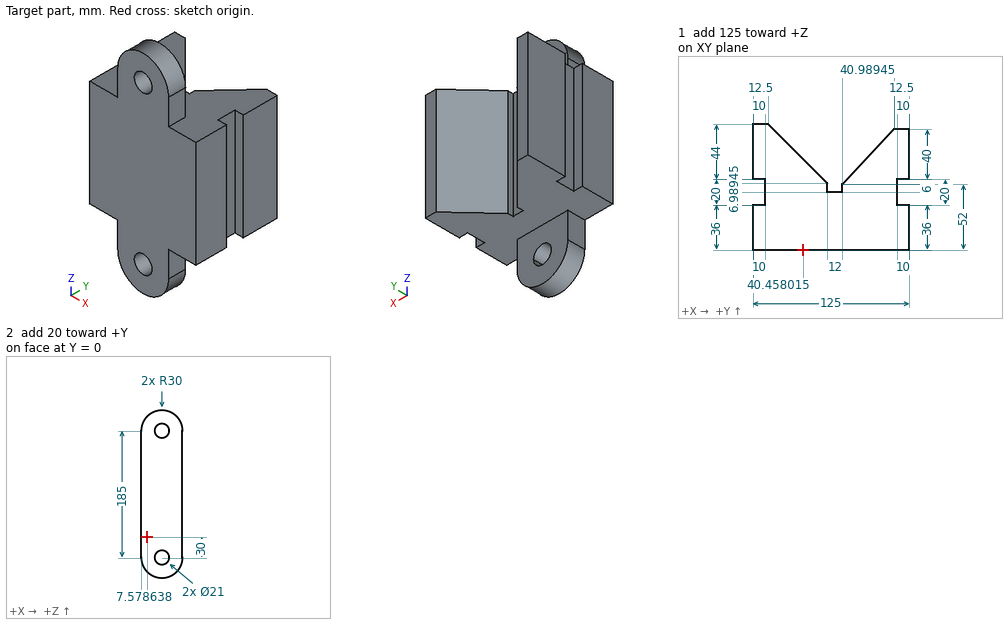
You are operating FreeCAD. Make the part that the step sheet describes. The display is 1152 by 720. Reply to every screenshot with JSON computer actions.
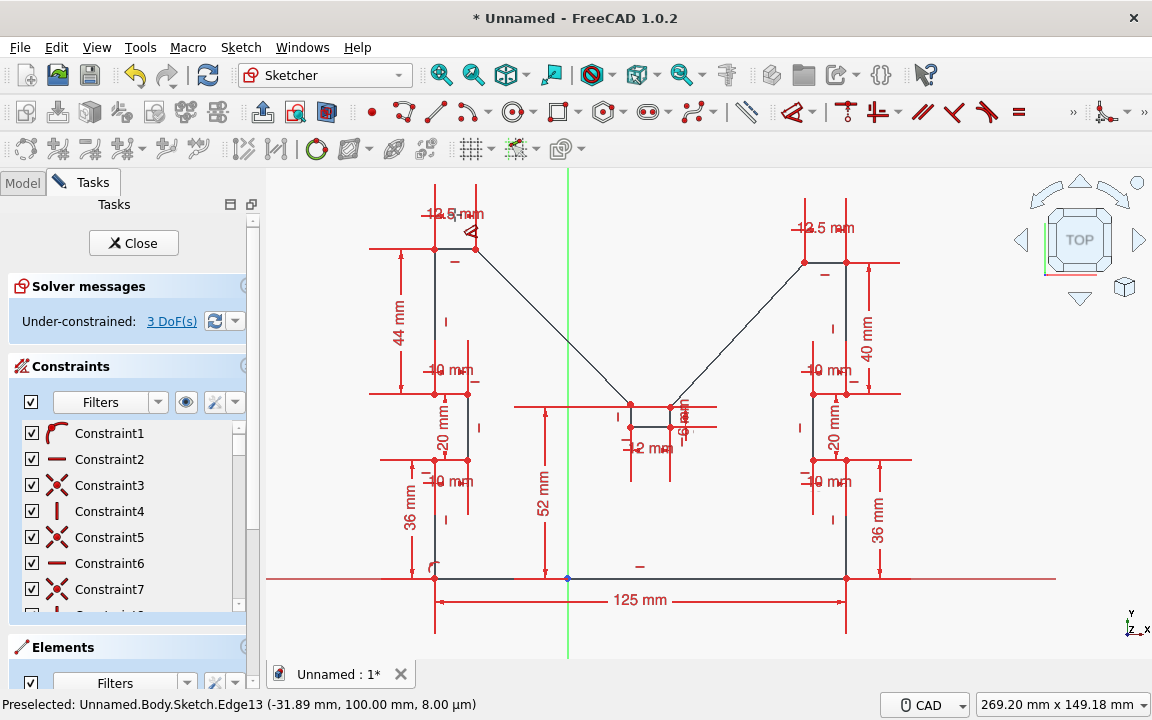
{"action": "scroll", "coordinate": [631, 416], "scroll_direction": "up", "scroll_amount": 3}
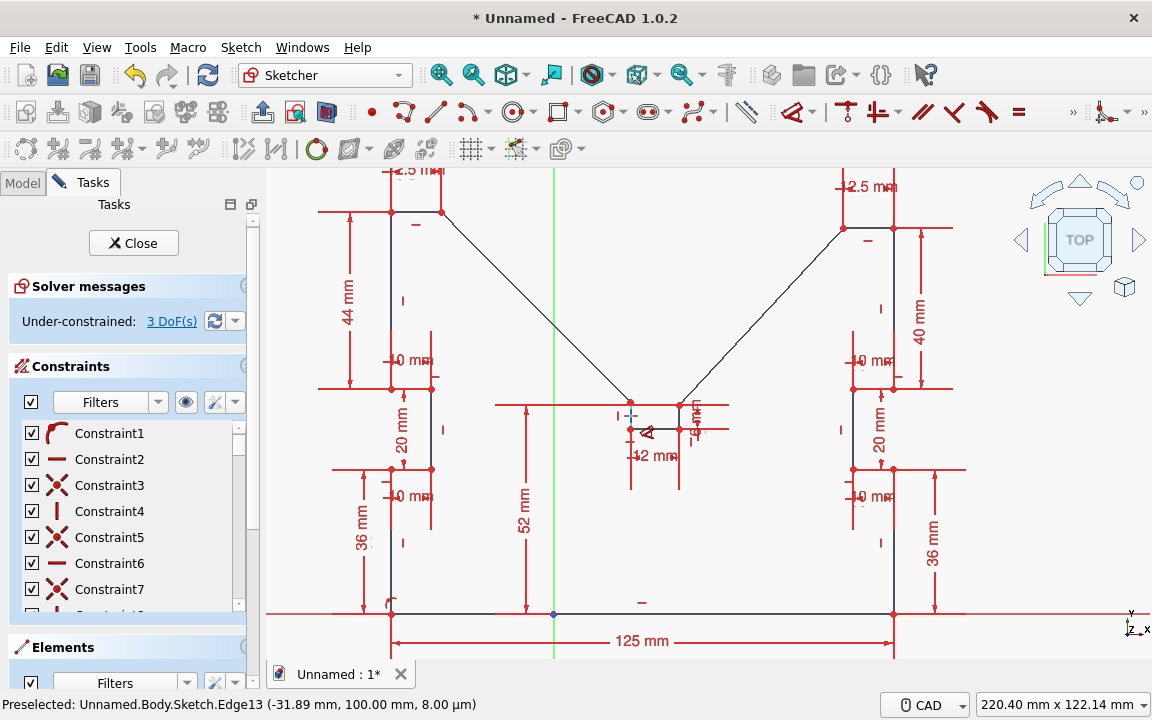
{"action": "left_click", "coordinate": [630, 416]}
{"action": "left_click", "coordinate": [596, 416]}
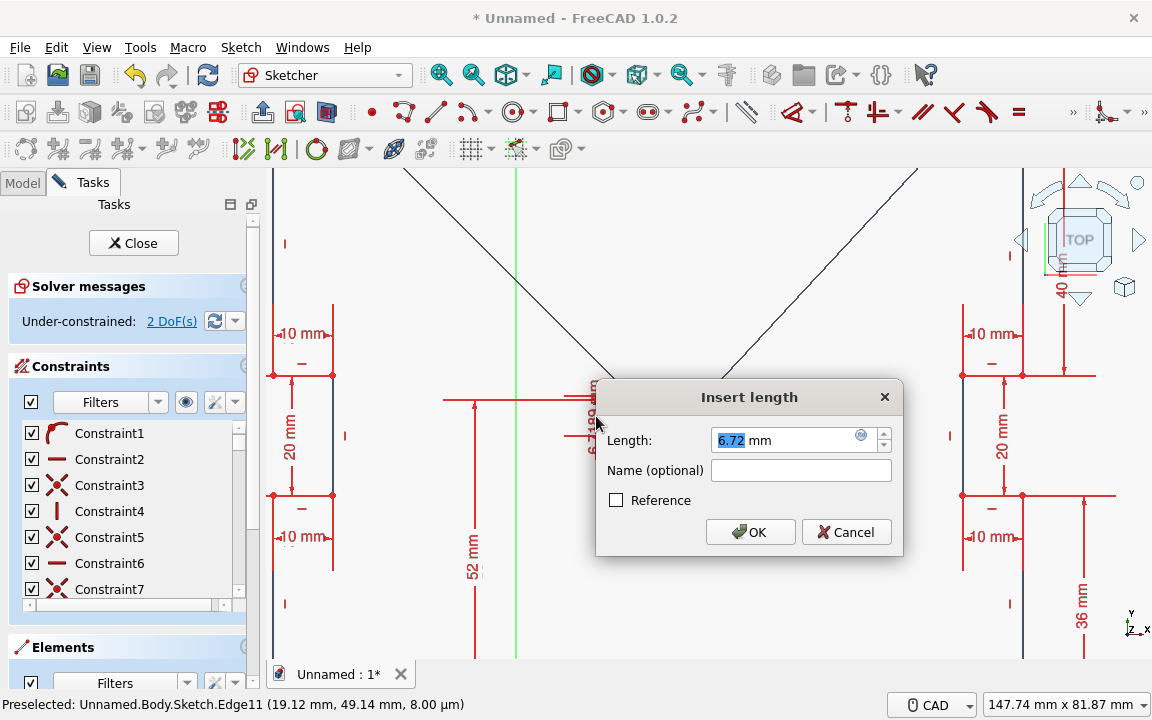
{"action": "type", "text": "6.98945"}
{"action": "key", "text": "Return"}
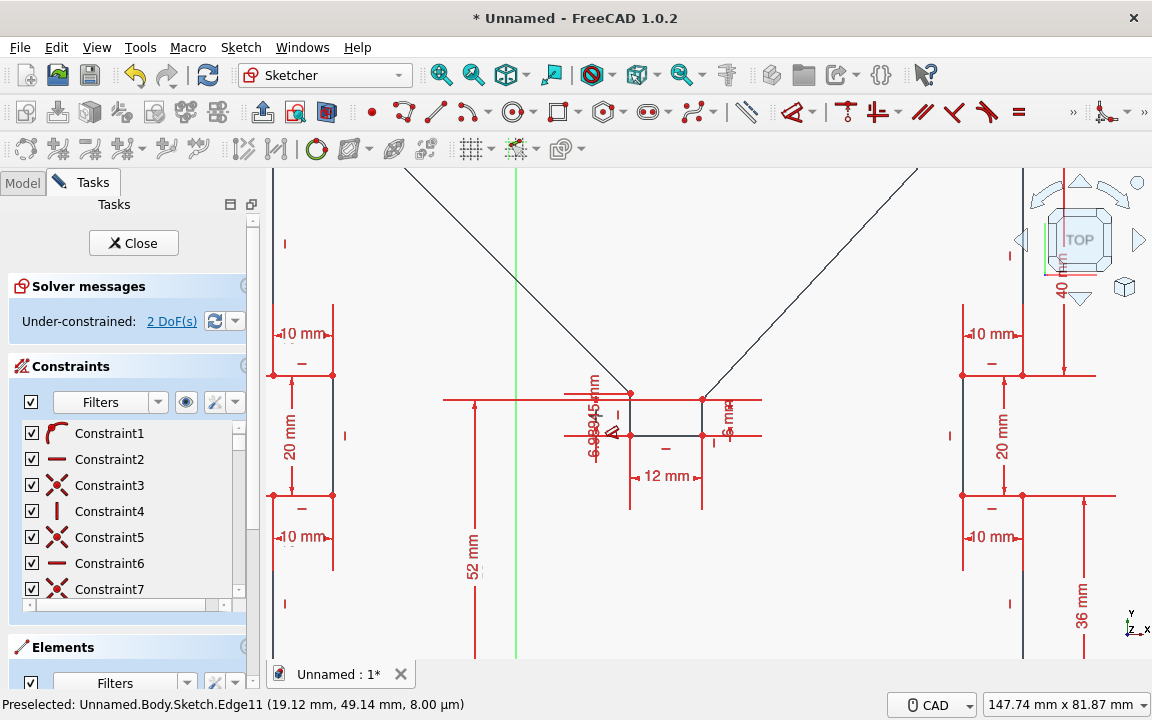
{"action": "left_click", "coordinate": [874, 215]}
{"action": "left_click", "coordinate": [825, 434]}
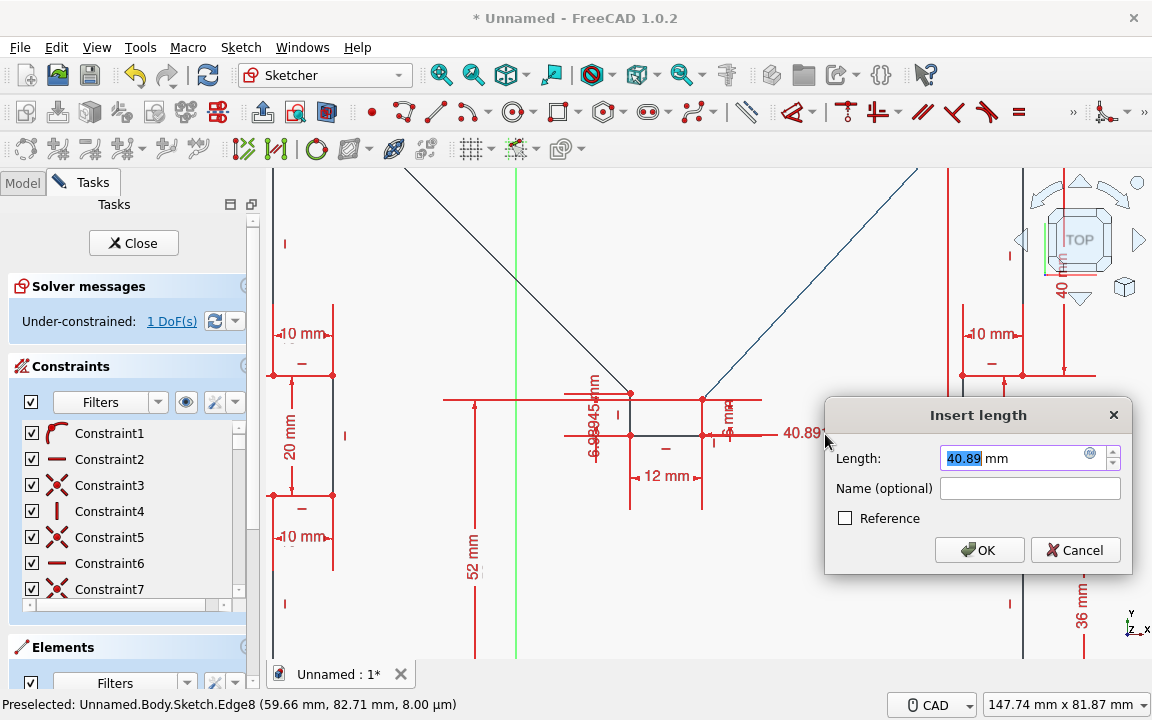
{"action": "type", "text": "40.98945"}
{"action": "key", "text": "Return"}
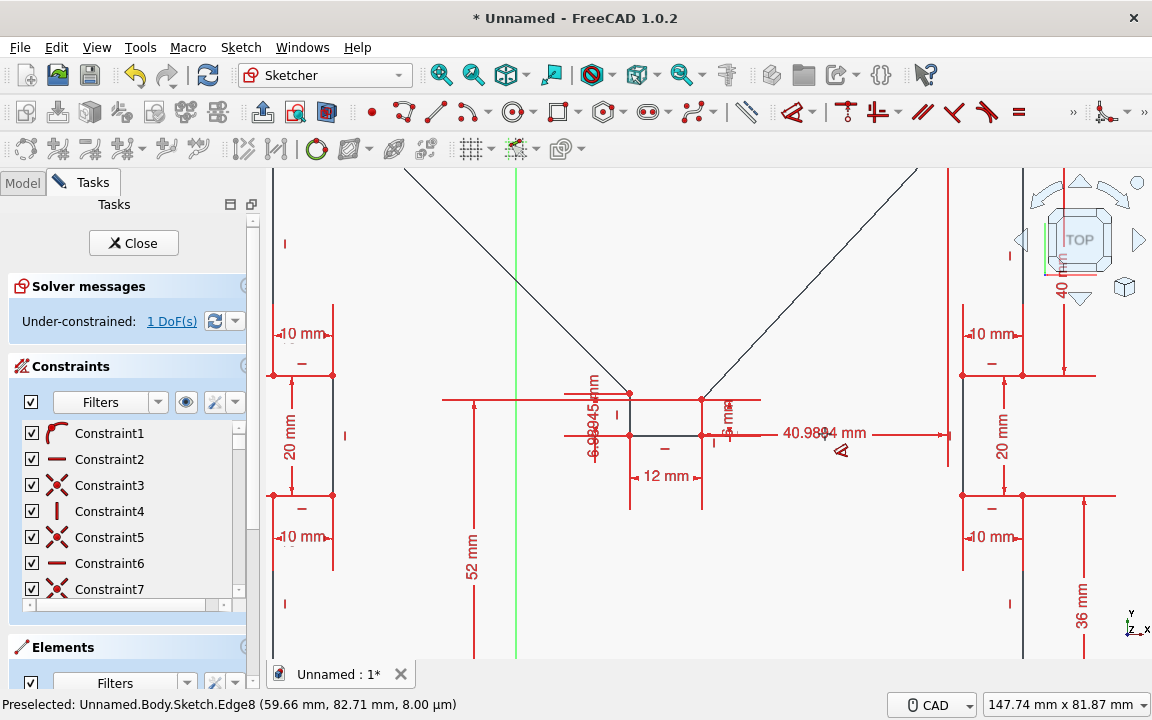
{"action": "scroll", "coordinate": [631, 416], "scroll_direction": "down", "scroll_amount": 3}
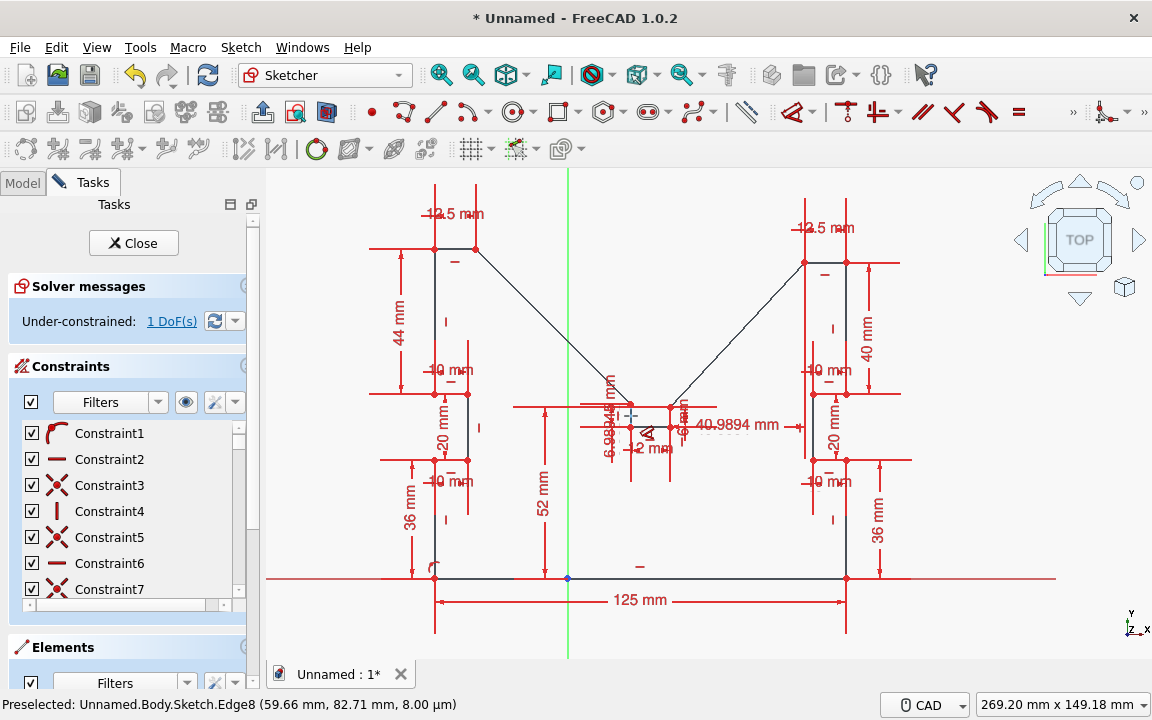
{"action": "left_click", "coordinate": [435, 579]}
{"action": "left_click", "coordinate": [501, 613]}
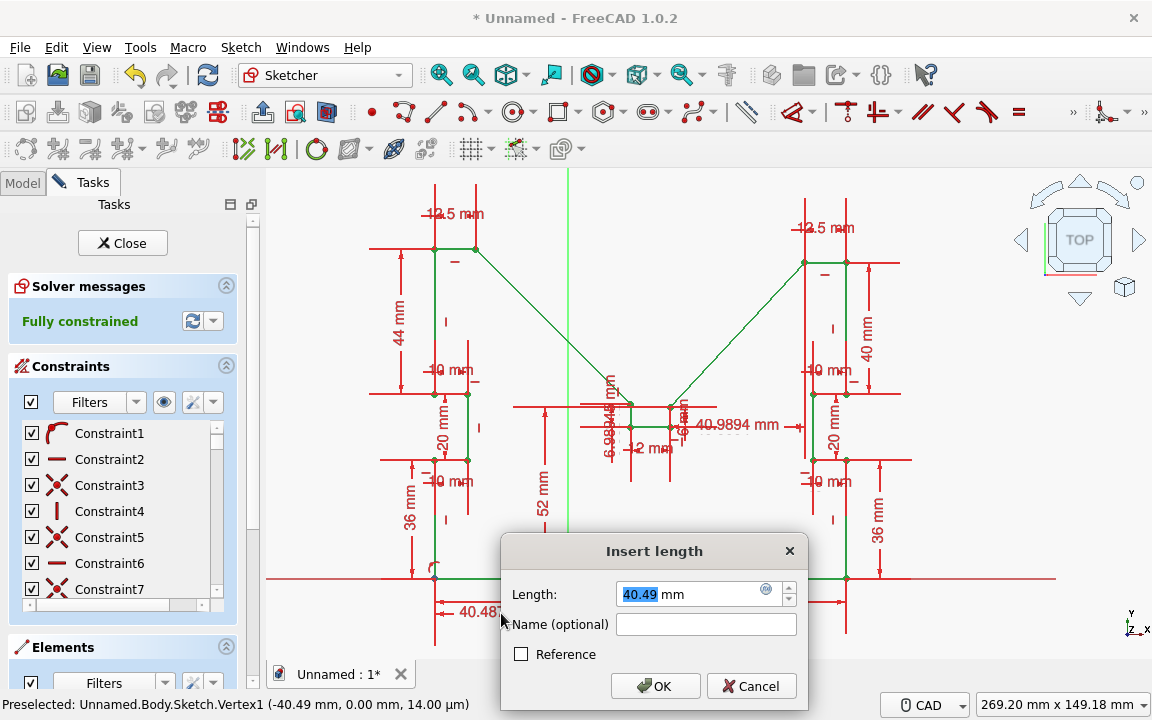
{"action": "type", "text": "40.458015"}
{"action": "key", "text": "Return"}
{"action": "key", "text": "Escape"}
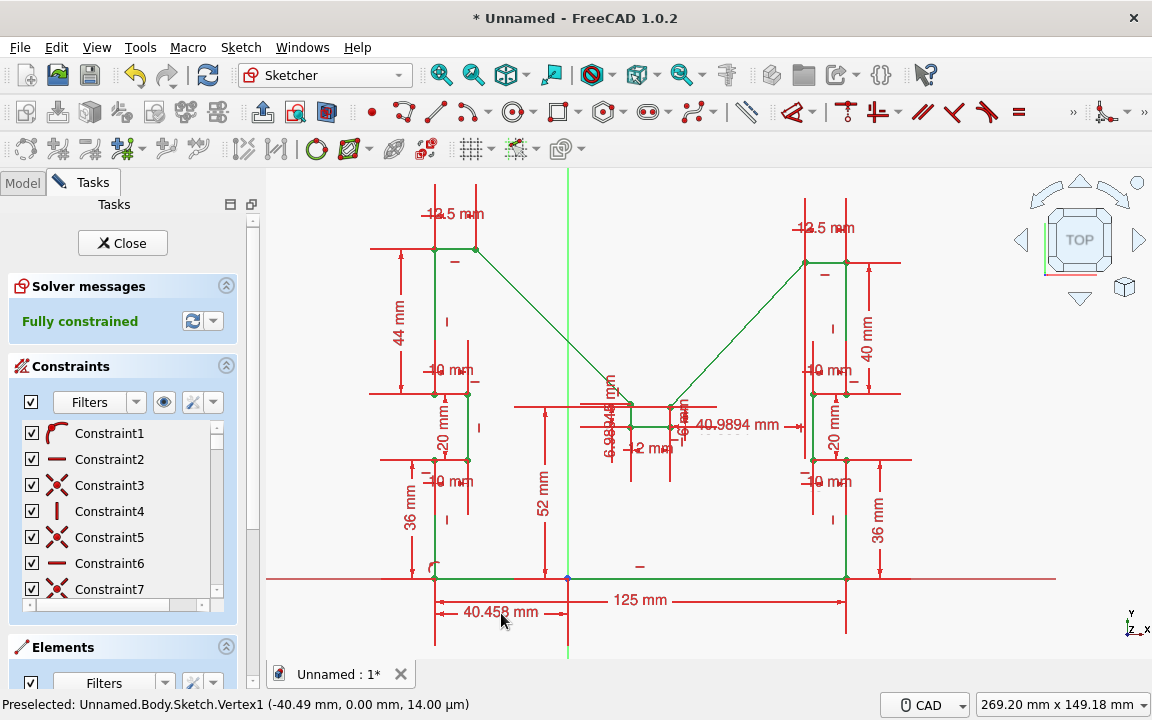
{"action": "left_click", "coordinate": [123, 243]}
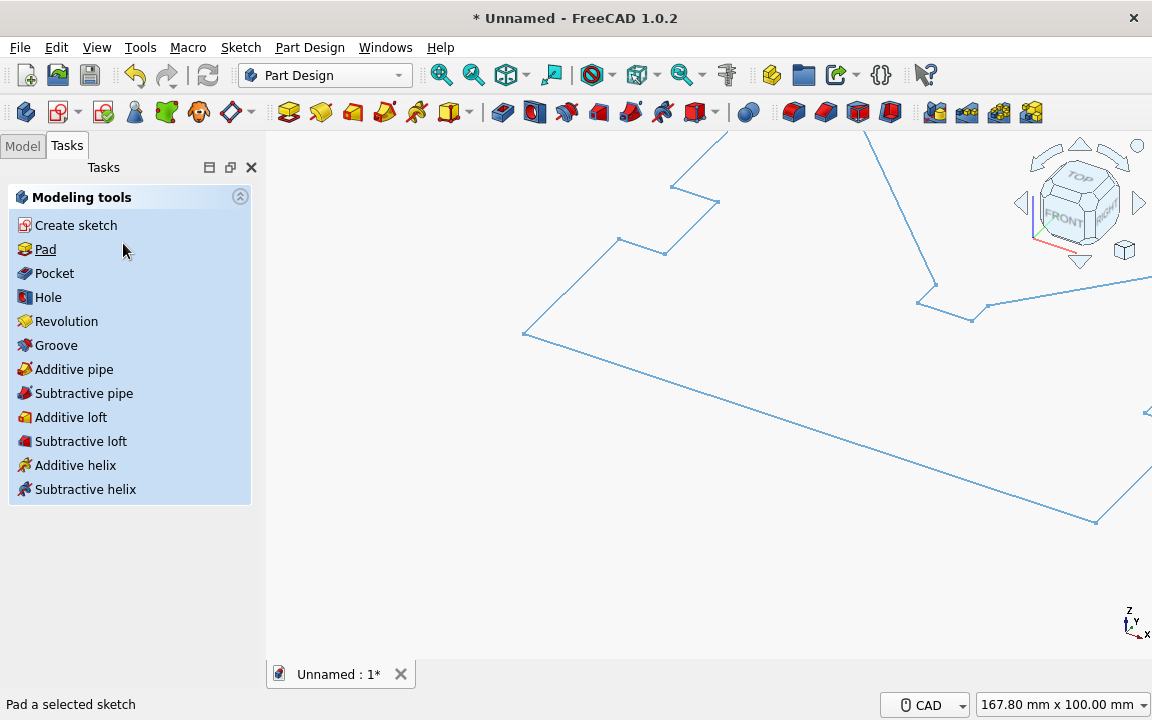
{"action": "left_click", "coordinate": [290, 112]}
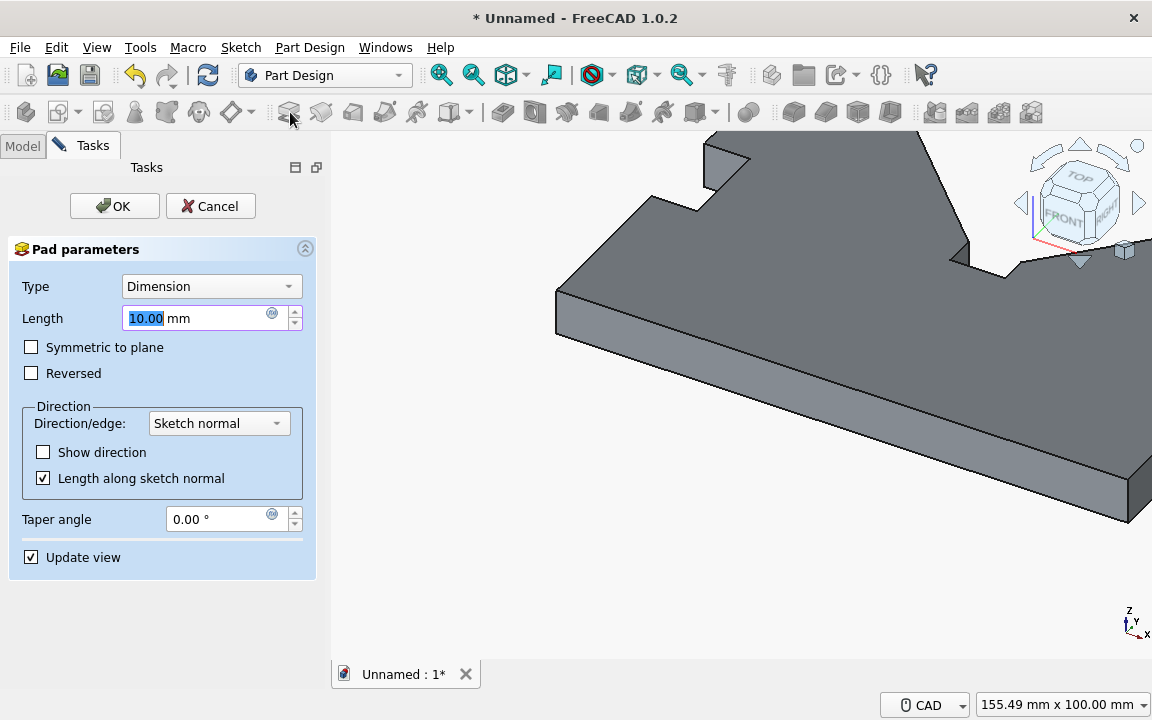
{"action": "type", "text": "125"}
{"action": "key", "text": "Tab"}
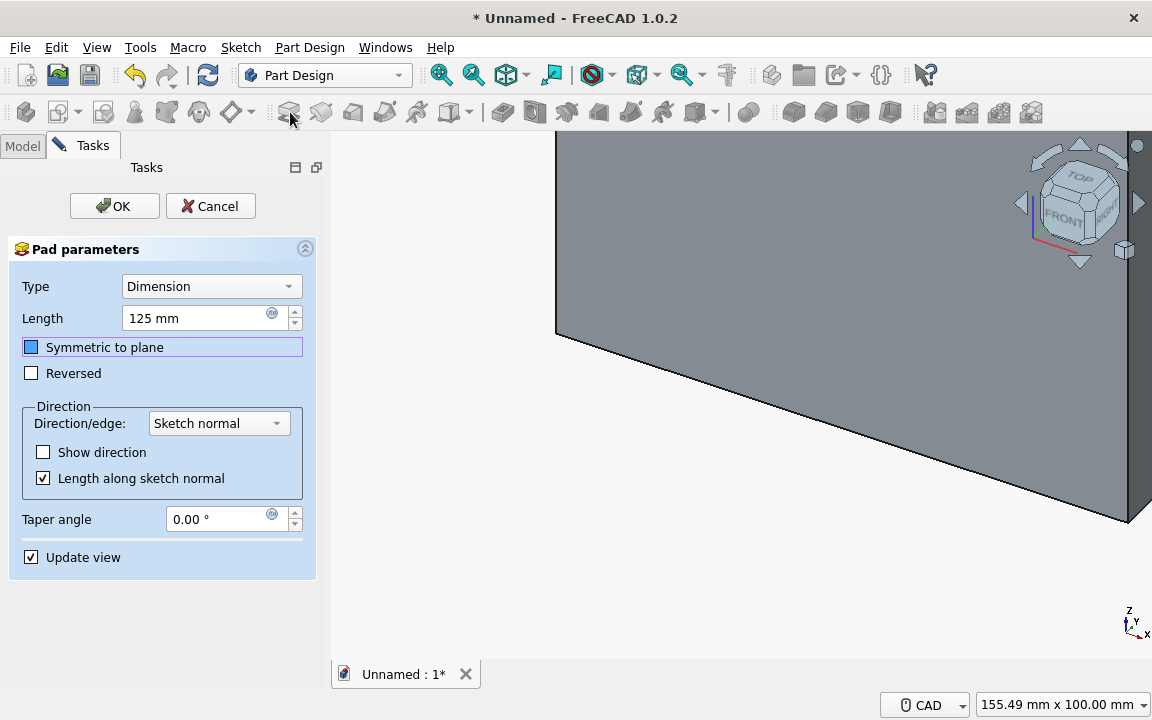
{"action": "left_click", "coordinate": [115, 206]}